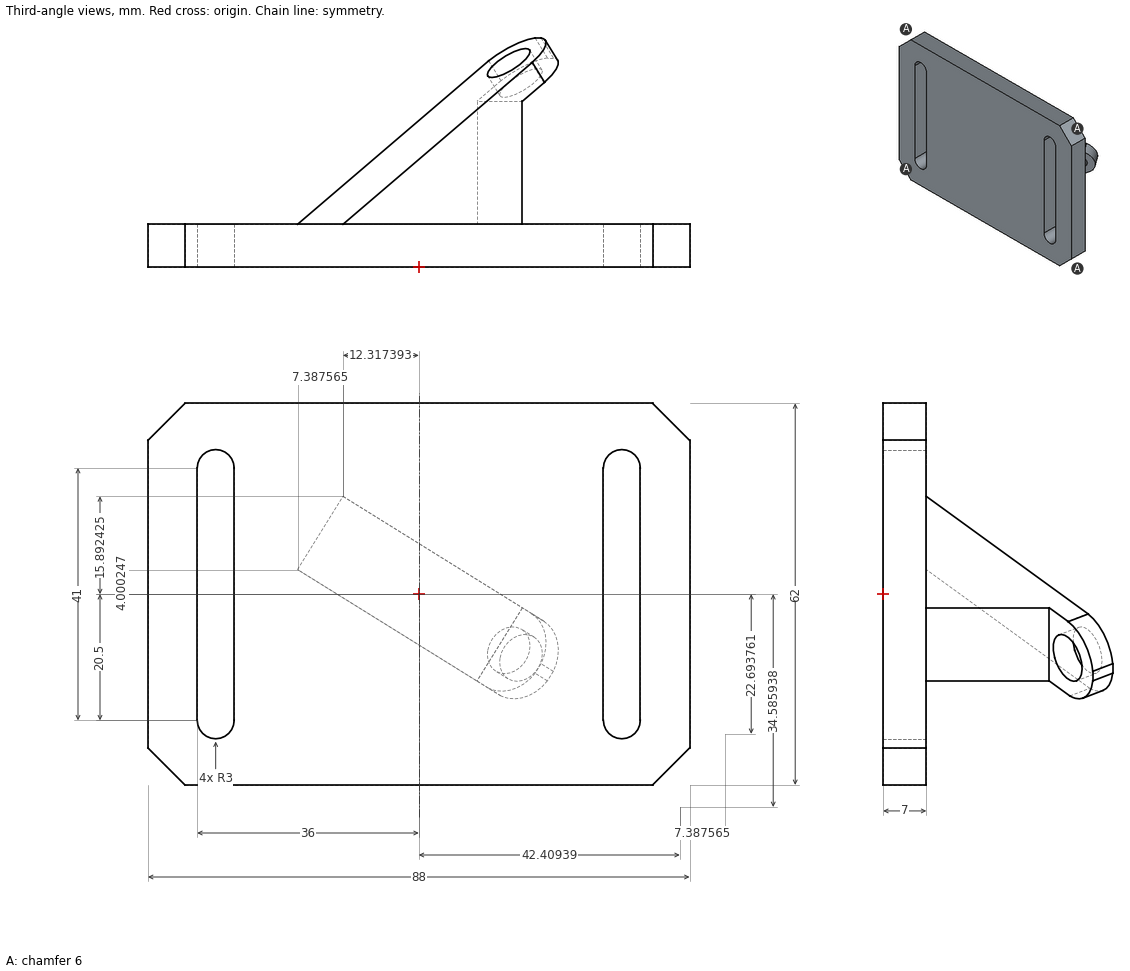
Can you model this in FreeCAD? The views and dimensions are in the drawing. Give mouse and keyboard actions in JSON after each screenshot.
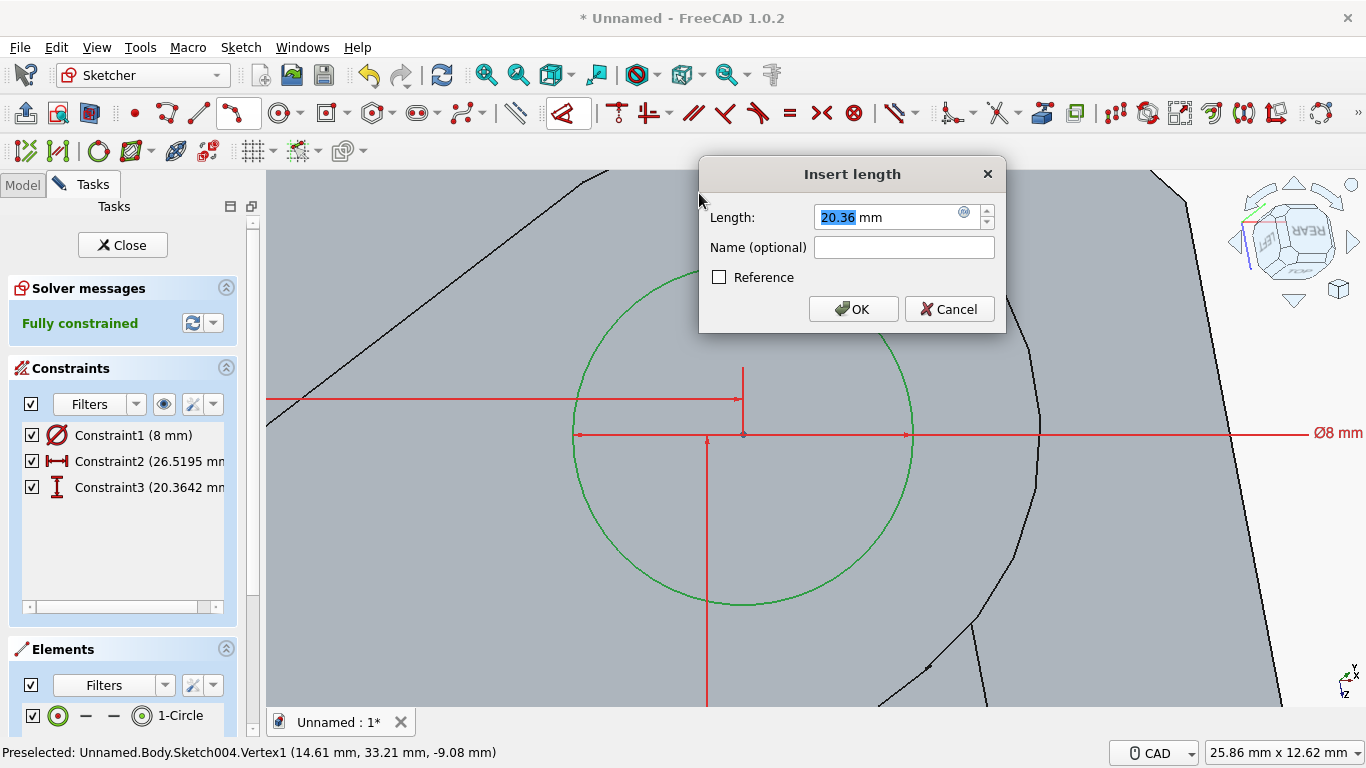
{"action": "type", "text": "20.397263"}
{"action": "key", "text": "Return"}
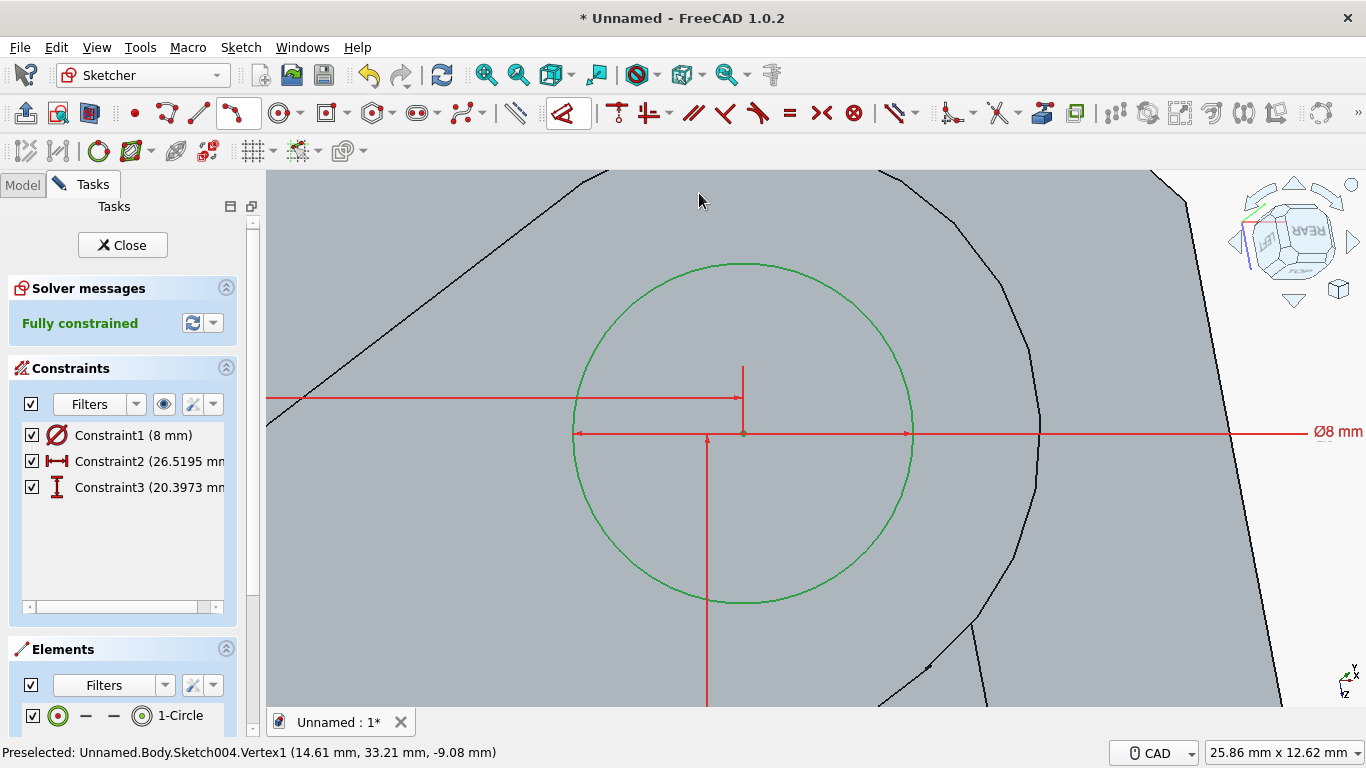
{"action": "left_click", "coordinate": [123, 245]}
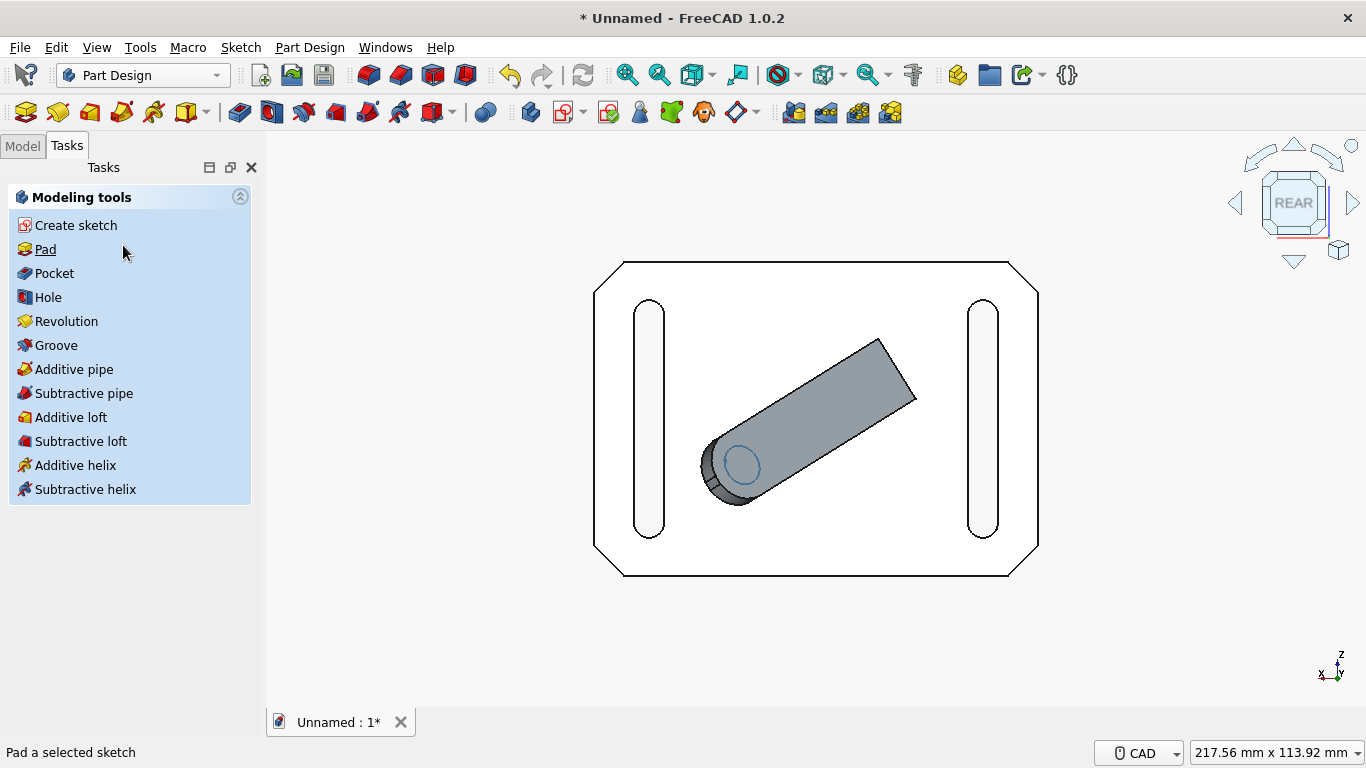
{"action": "left_click", "coordinate": [240, 112]}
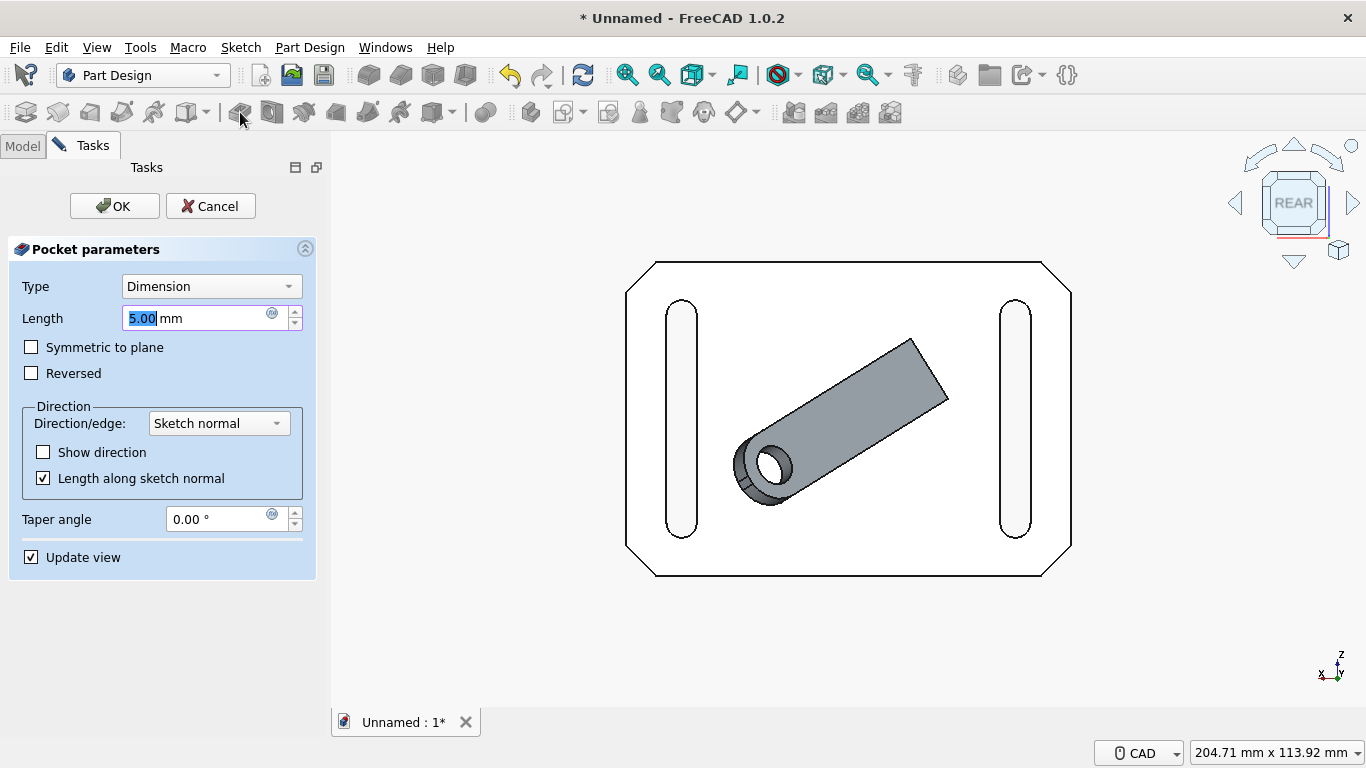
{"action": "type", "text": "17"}
{"action": "key", "text": "Tab"}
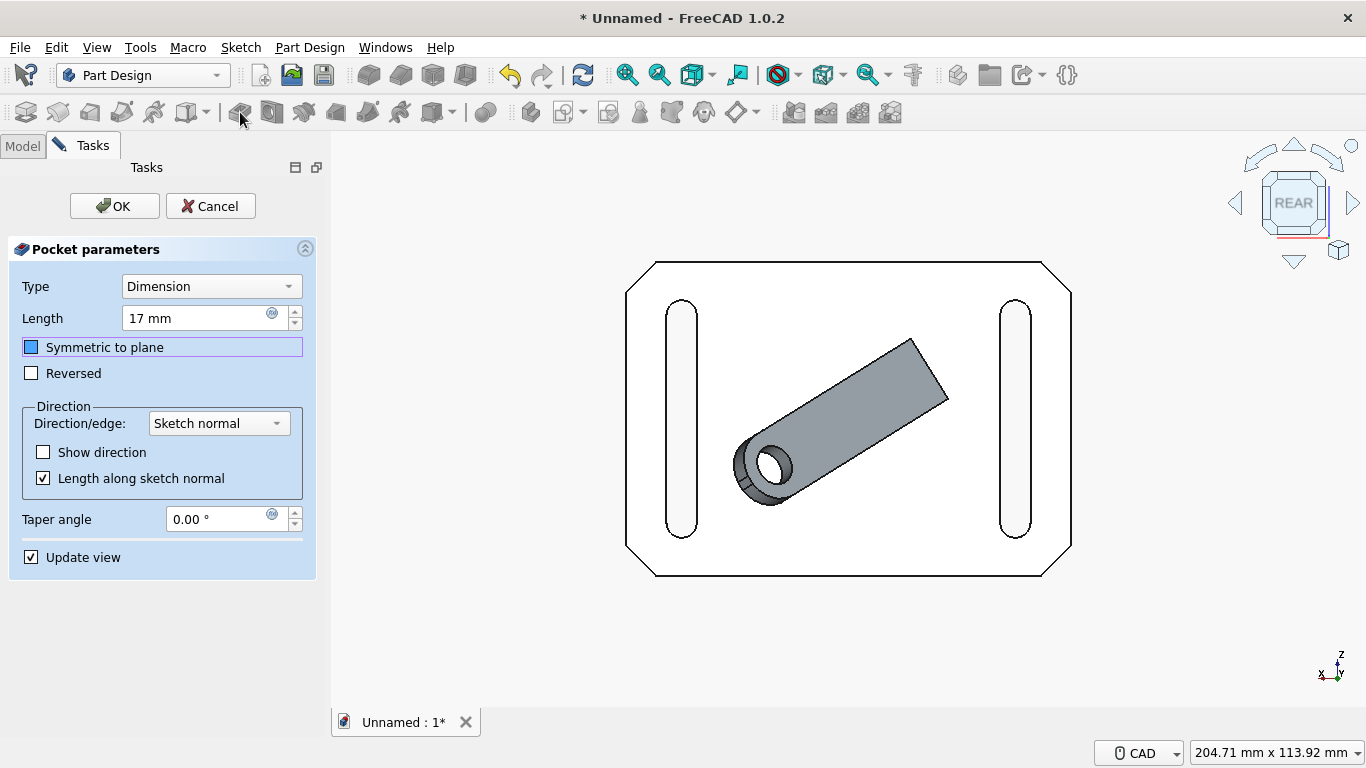
{"action": "left_click", "coordinate": [115, 206]}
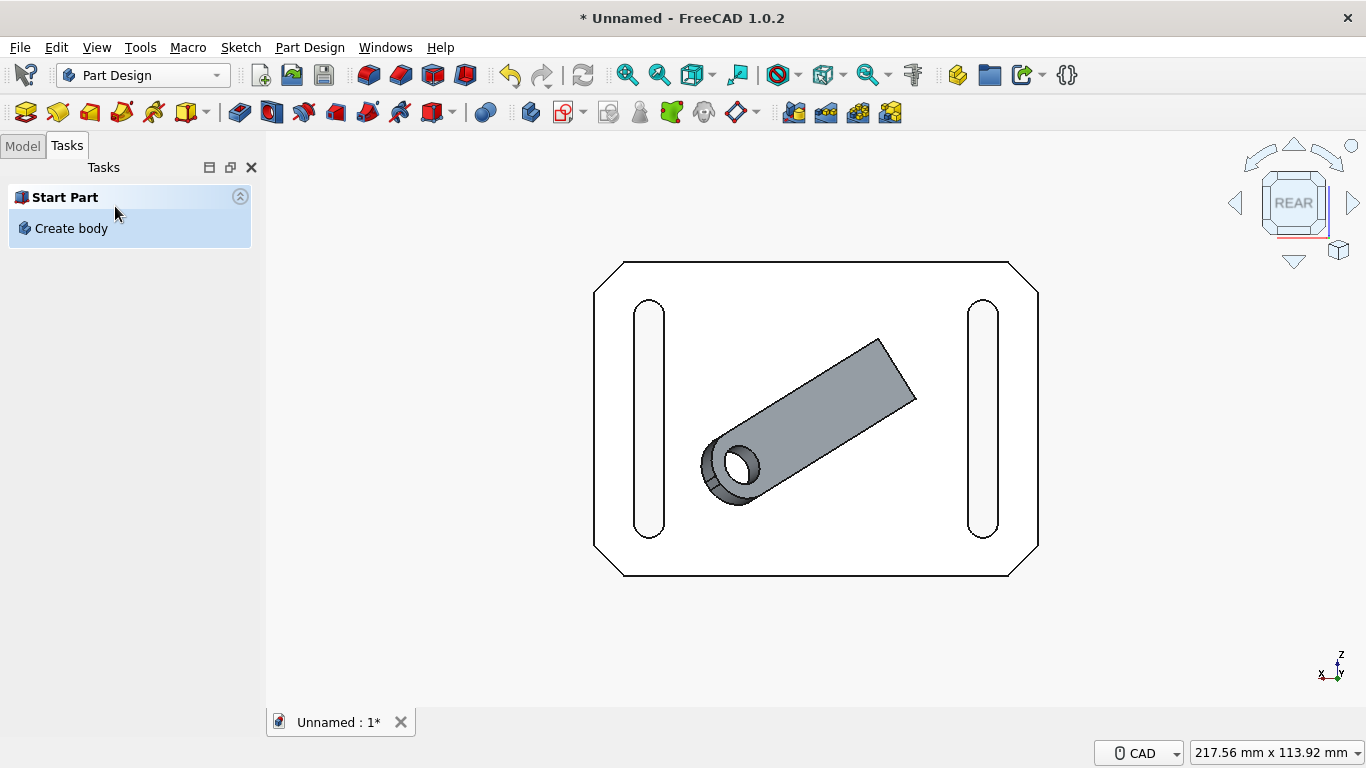
{"action": "key", "text": "0"}